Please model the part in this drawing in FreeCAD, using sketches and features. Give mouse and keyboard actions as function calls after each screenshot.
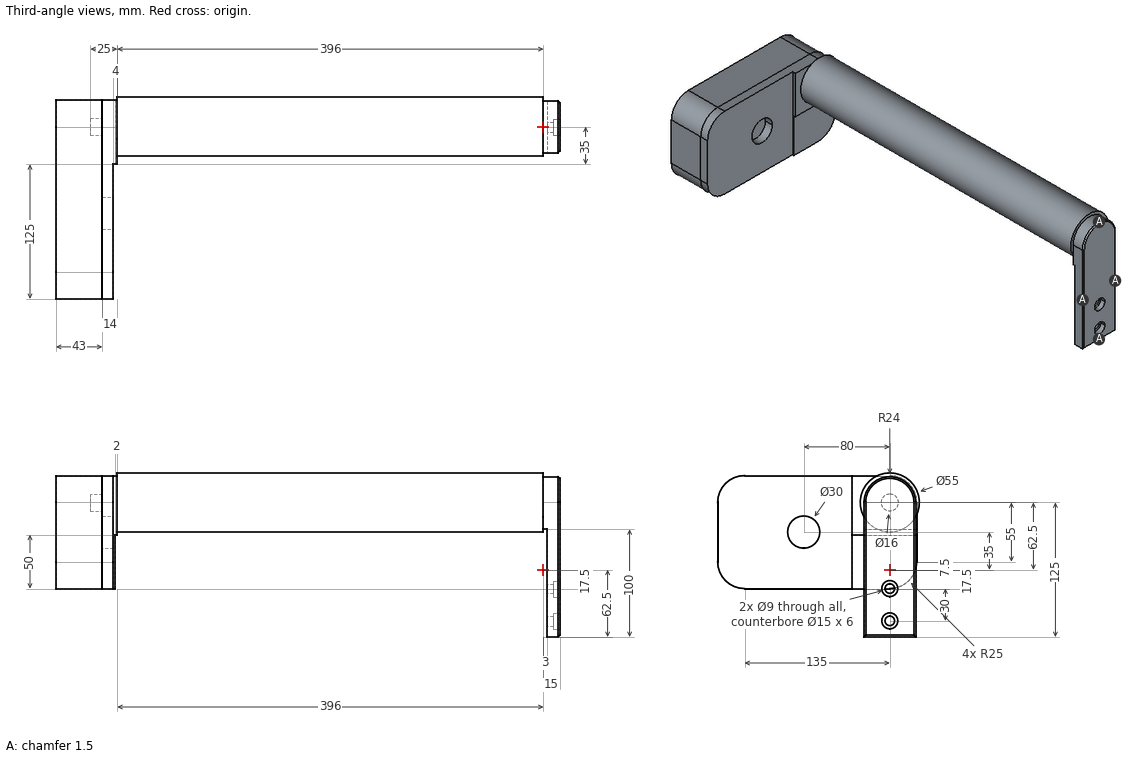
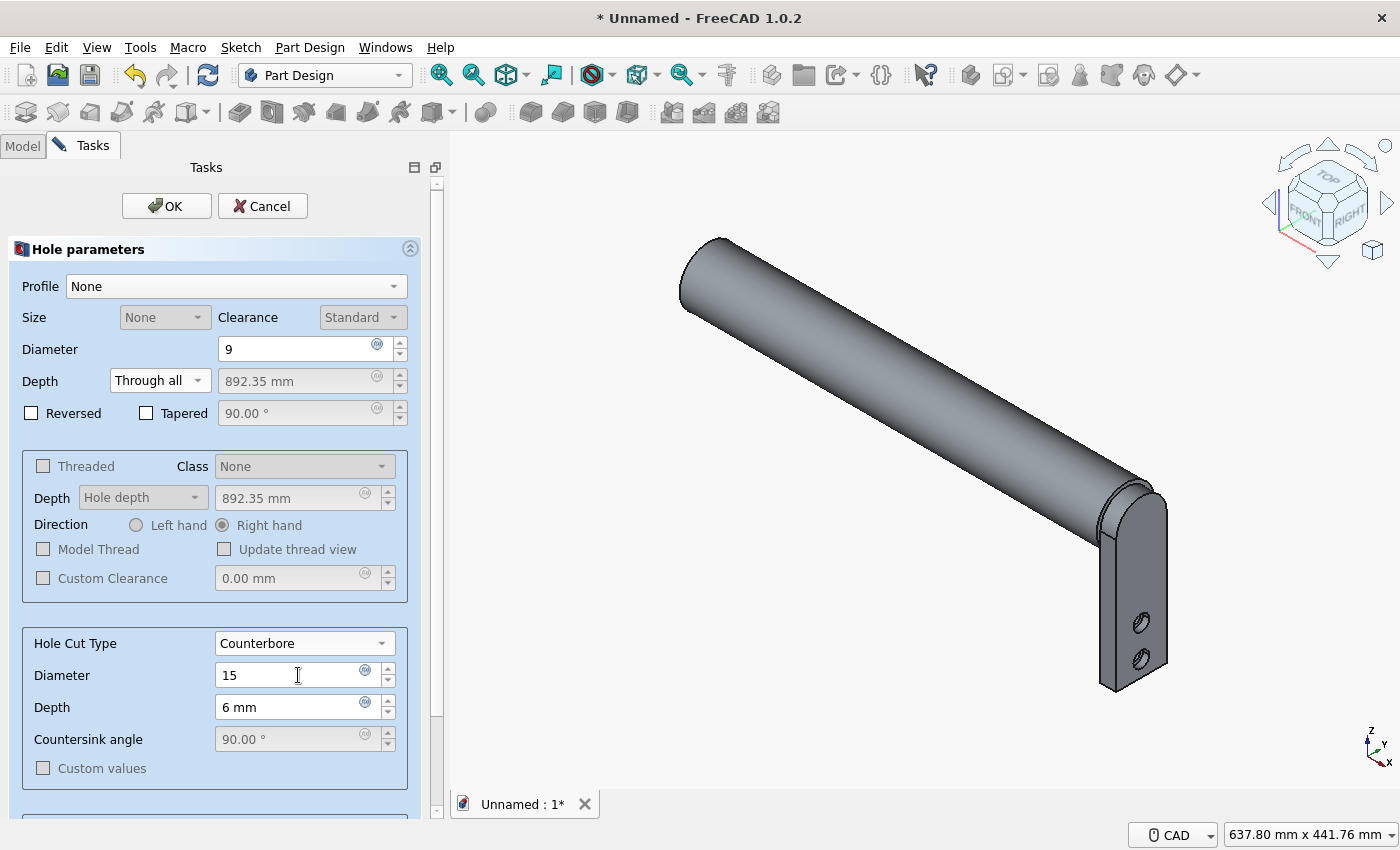
click(167, 206)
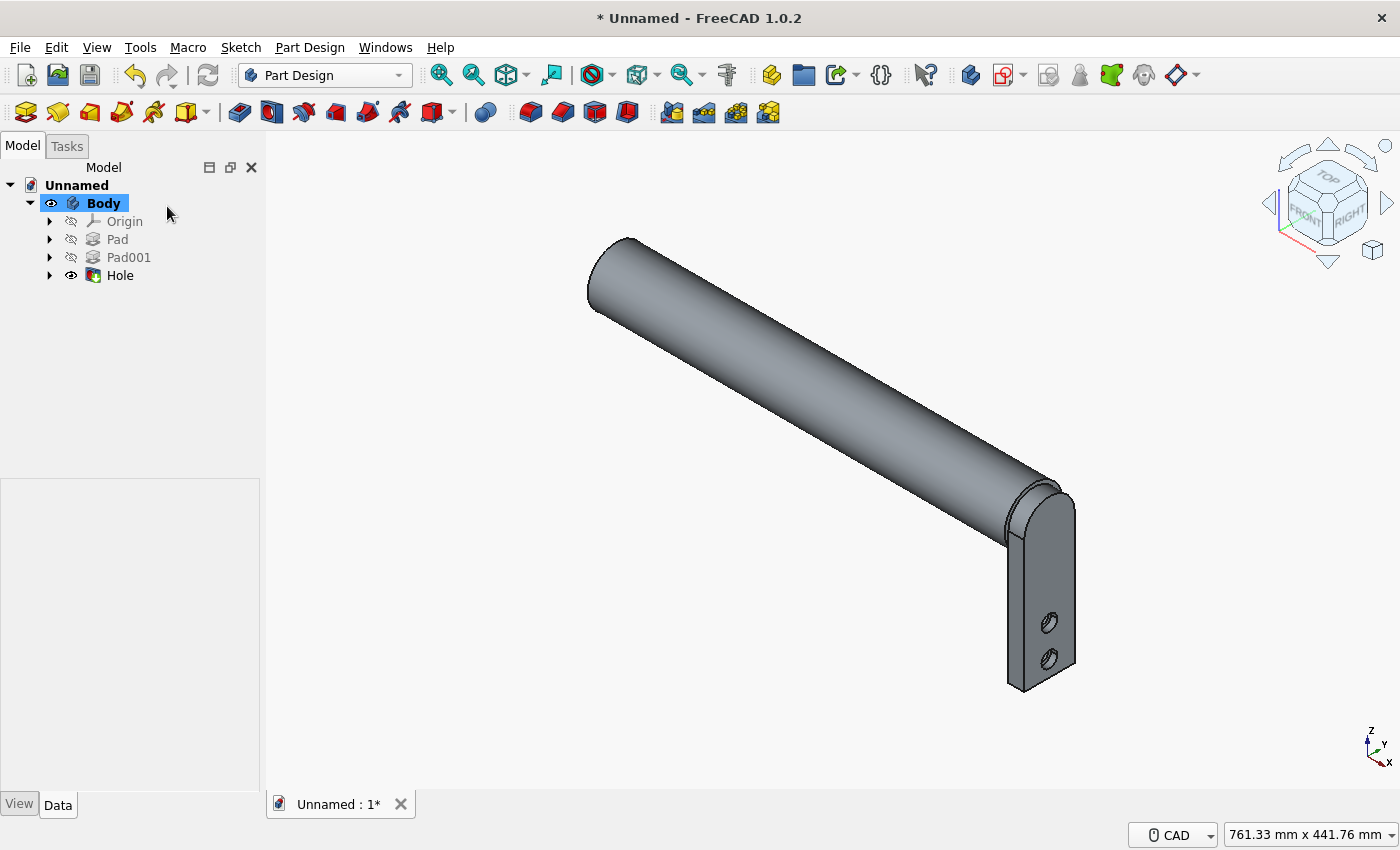
click(1049, 495)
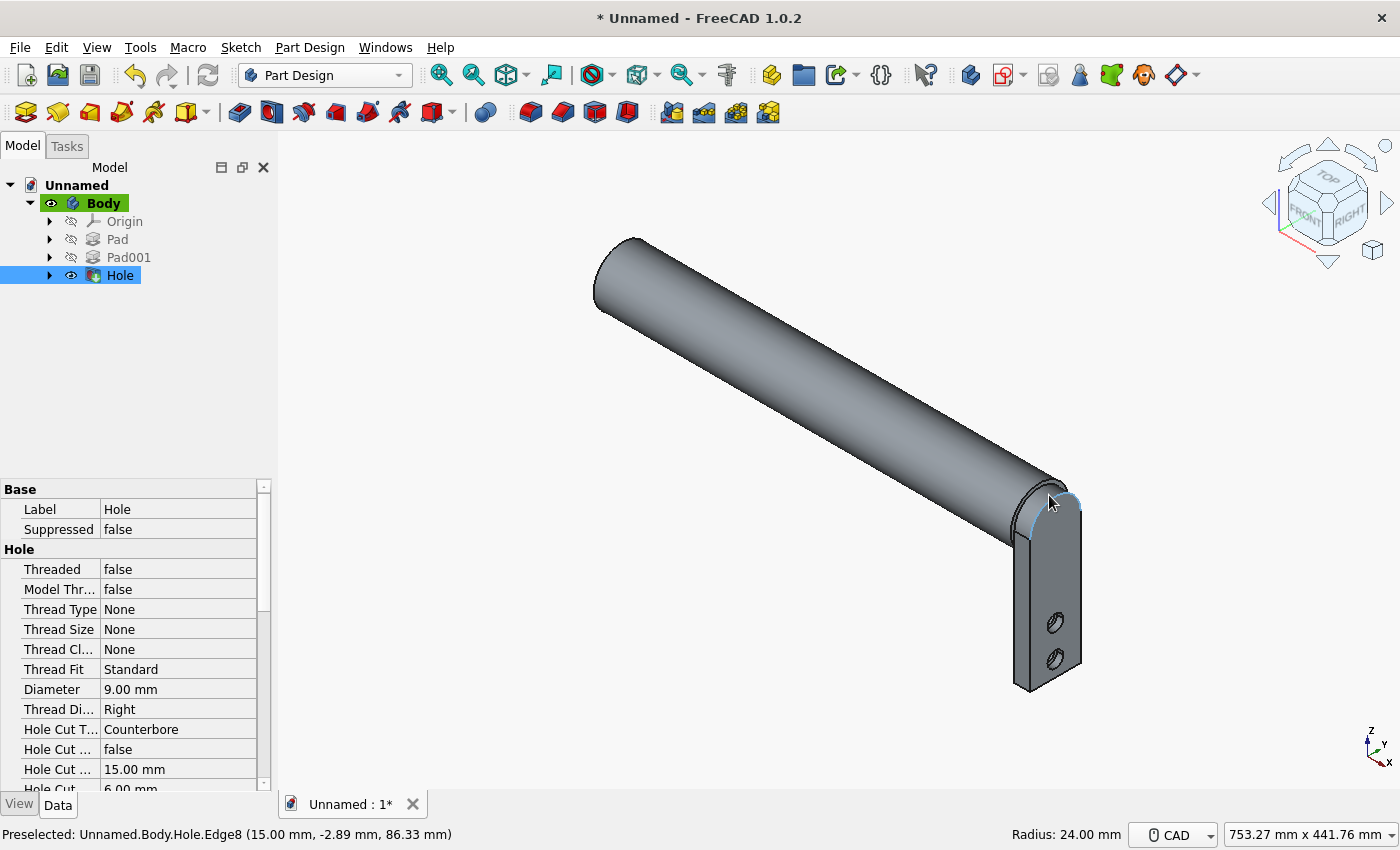
click(1030, 615, ctrl)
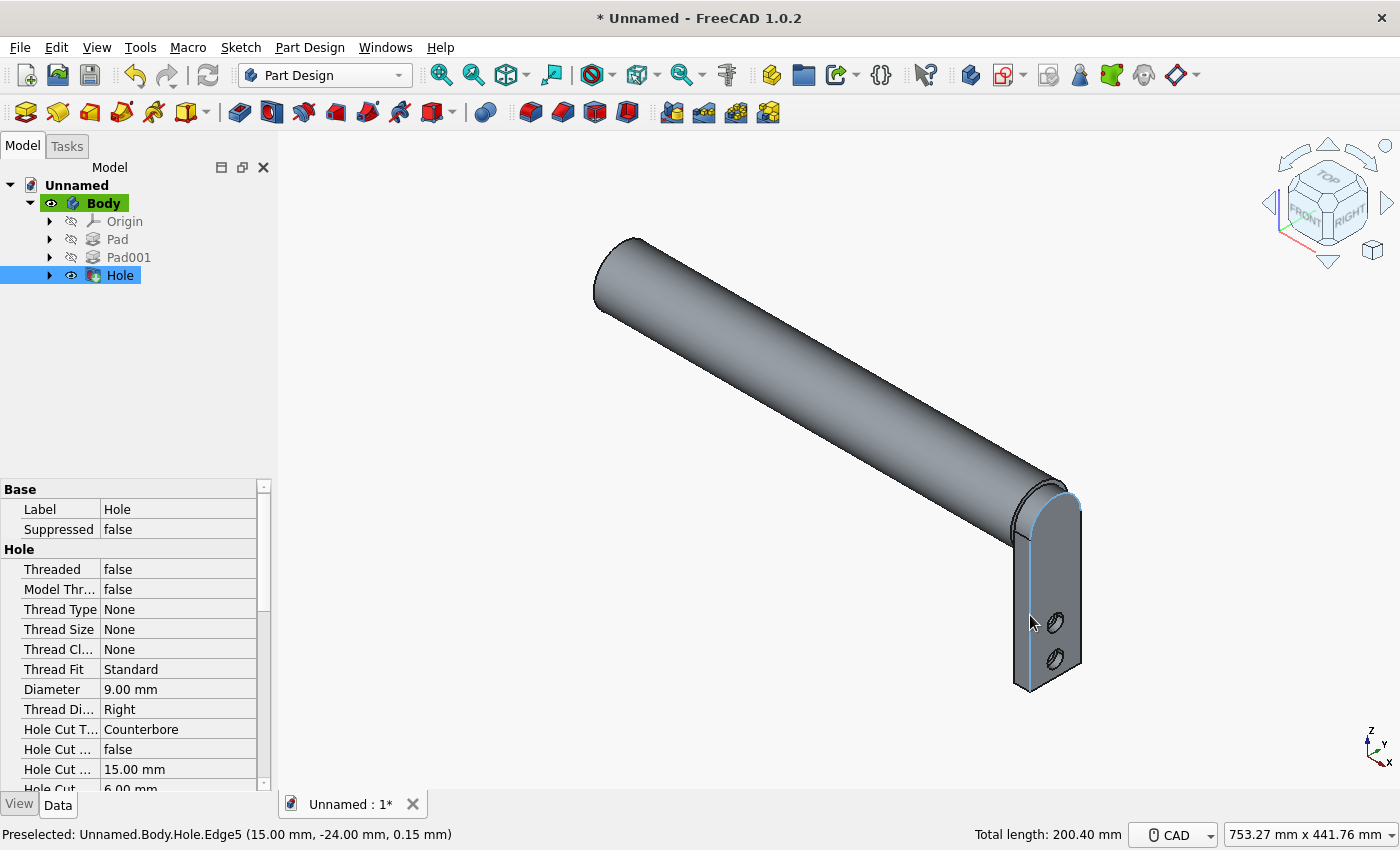
key(2)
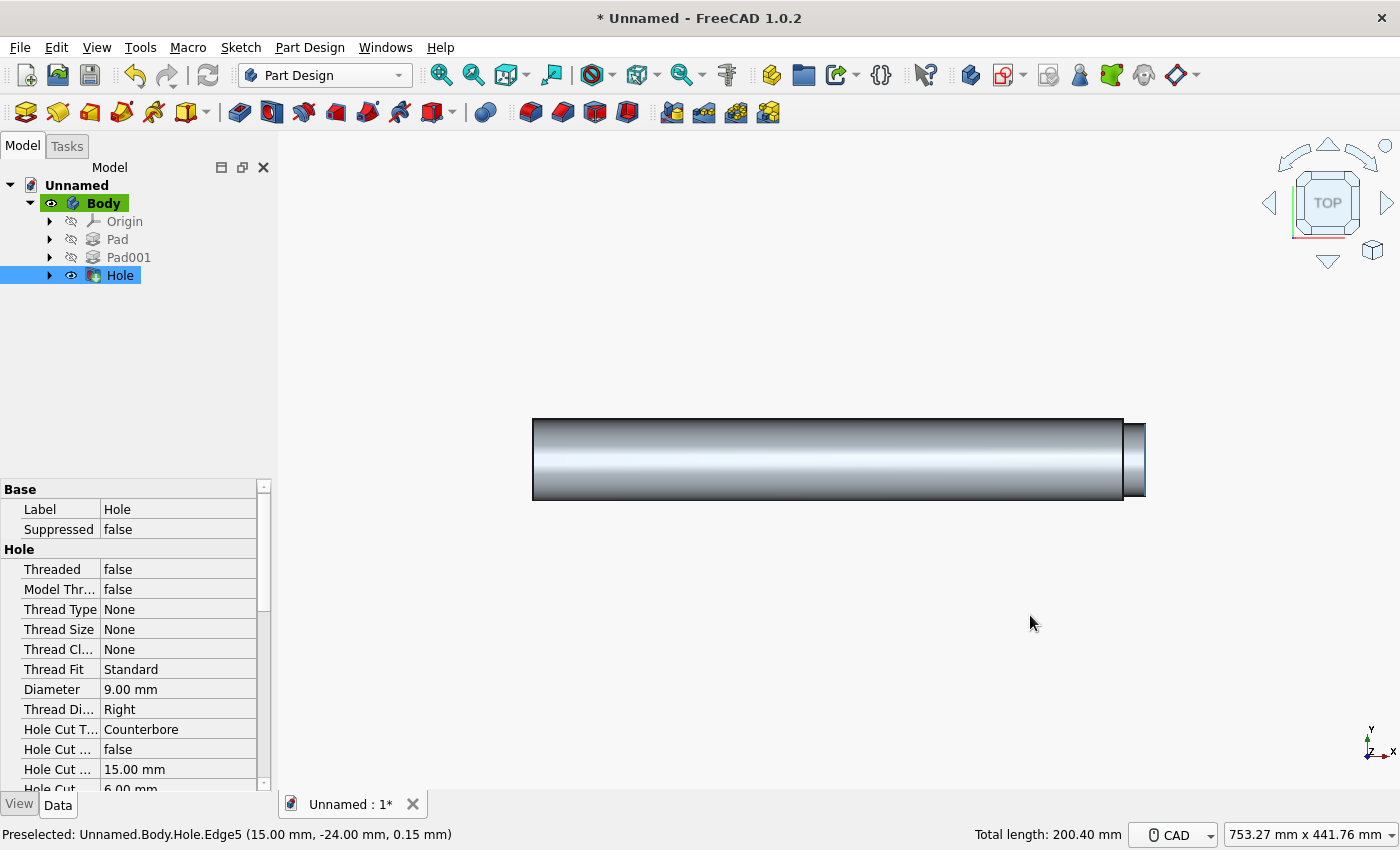
key(0)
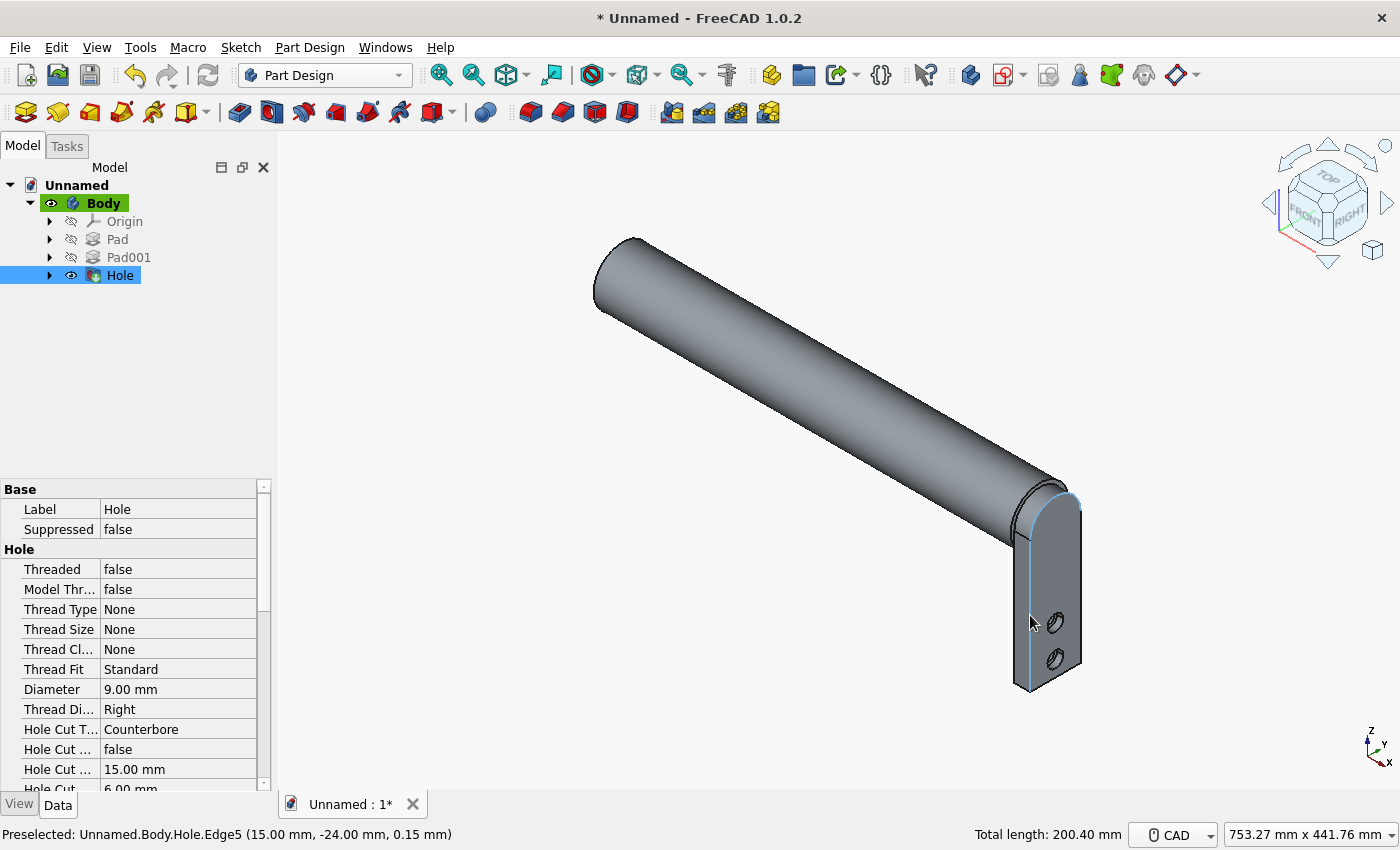
key(1)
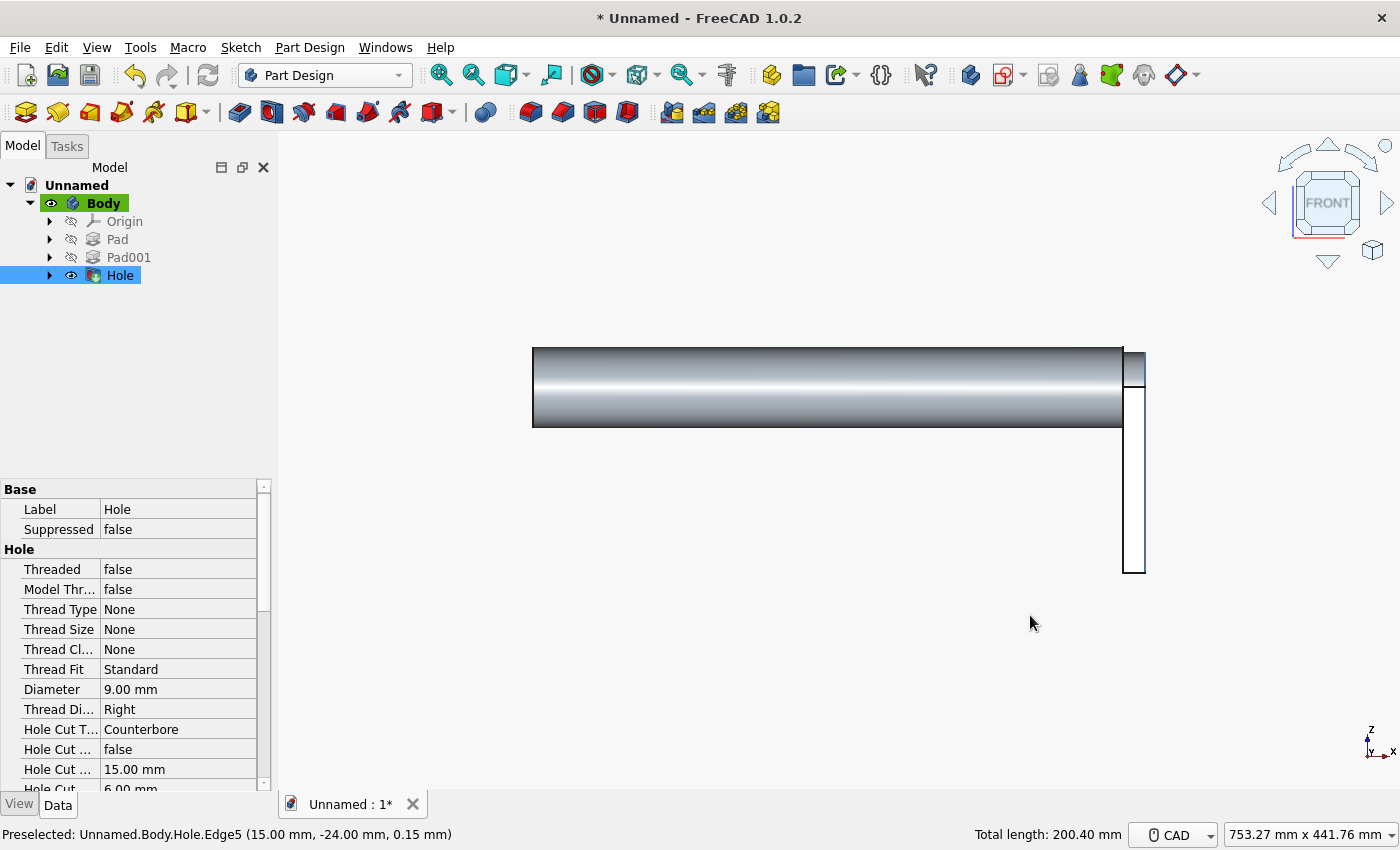
key(3)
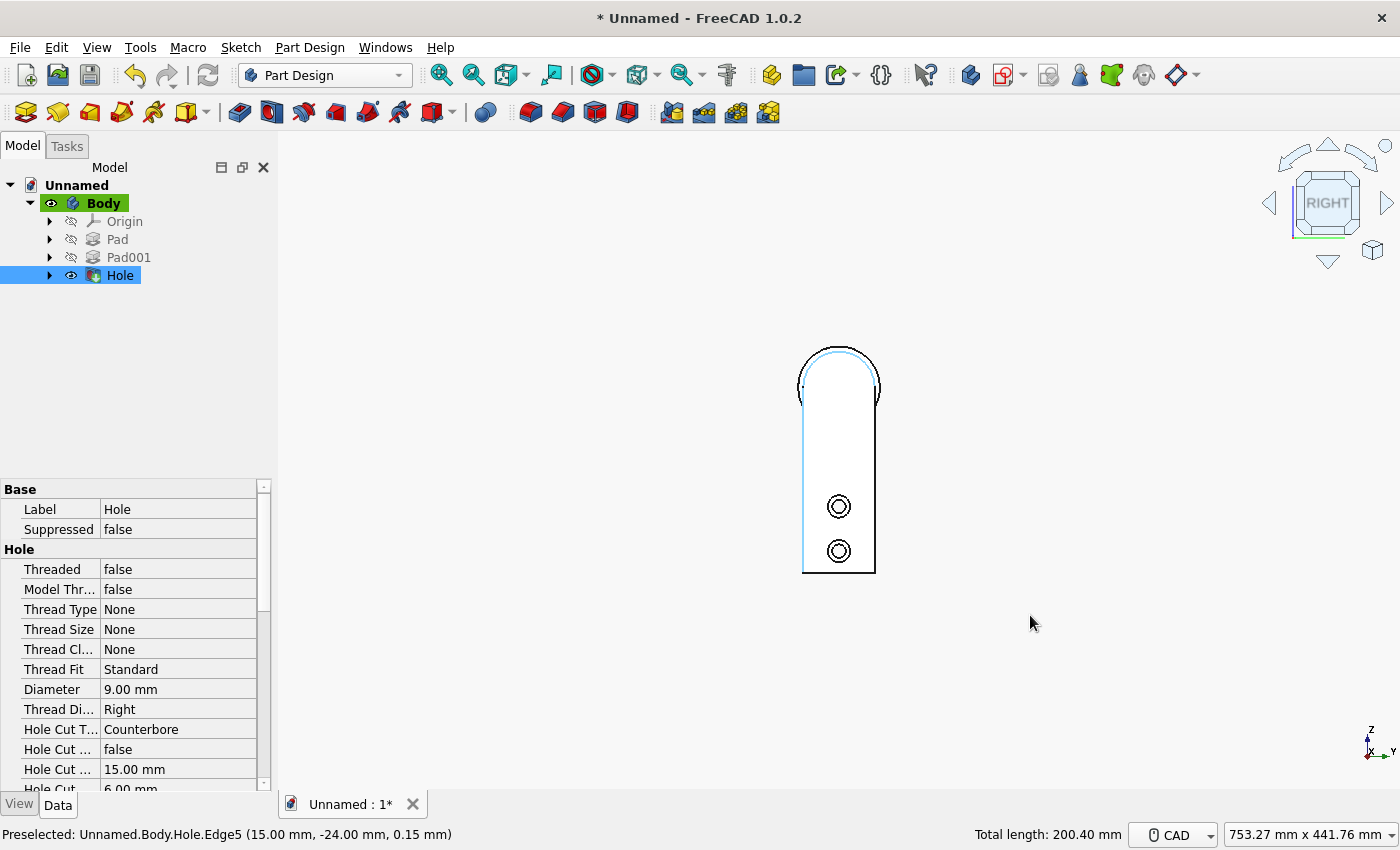
click(442, 76)